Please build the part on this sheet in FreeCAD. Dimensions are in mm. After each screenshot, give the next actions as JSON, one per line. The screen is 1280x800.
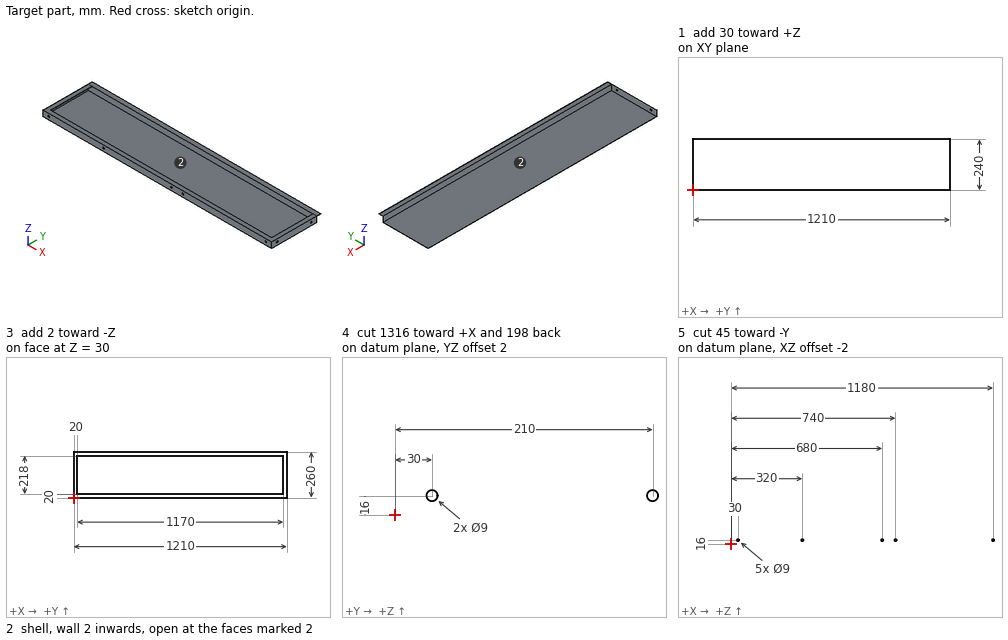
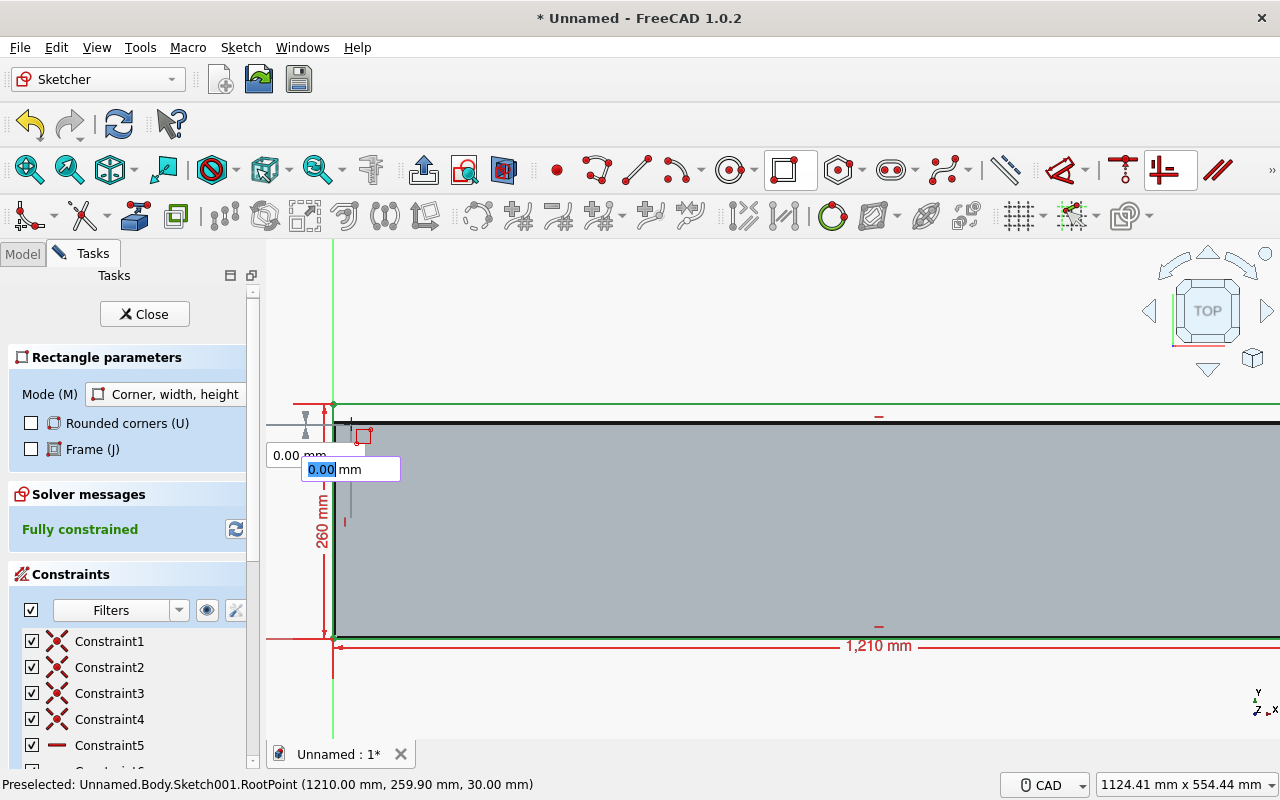
{"action": "scroll", "coordinate": [492, 449], "scroll_direction": "down", "scroll_amount": 3}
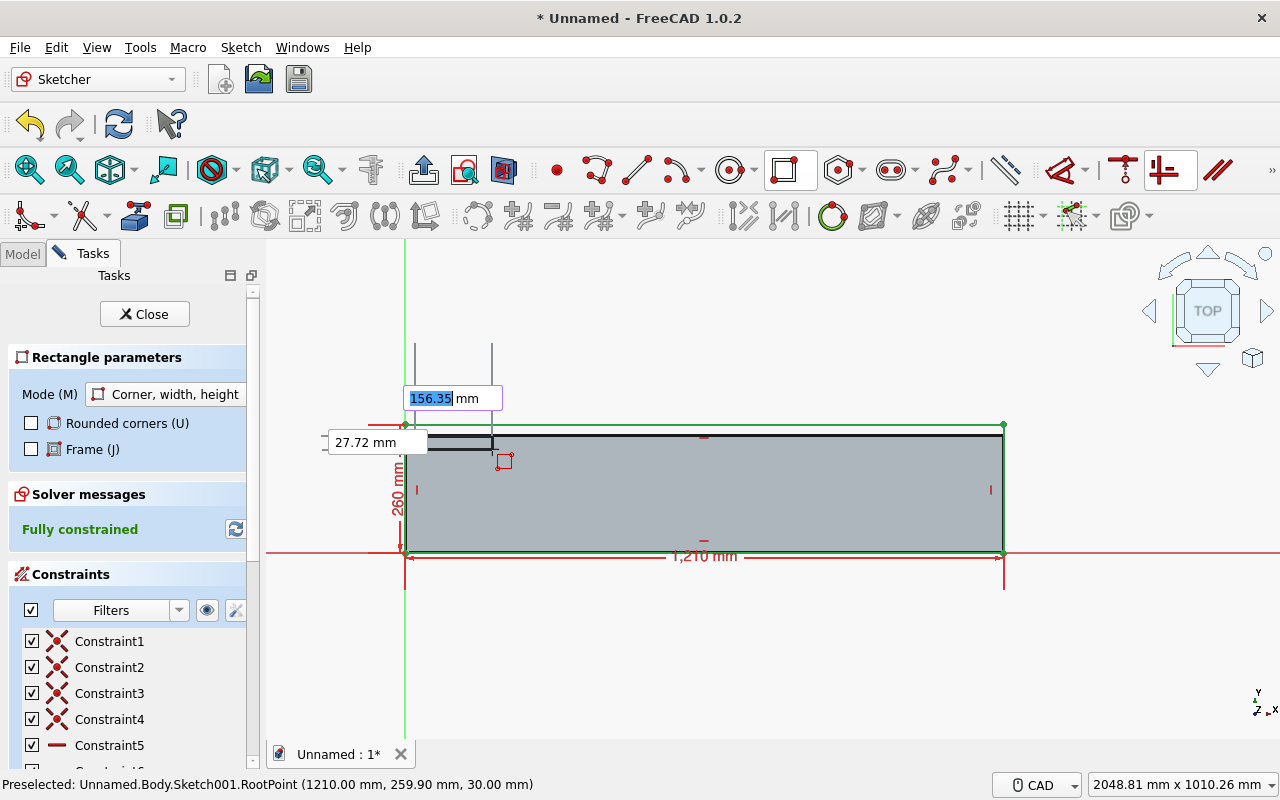
{"action": "scroll", "coordinate": [994, 543], "scroll_direction": "up", "scroll_amount": 3}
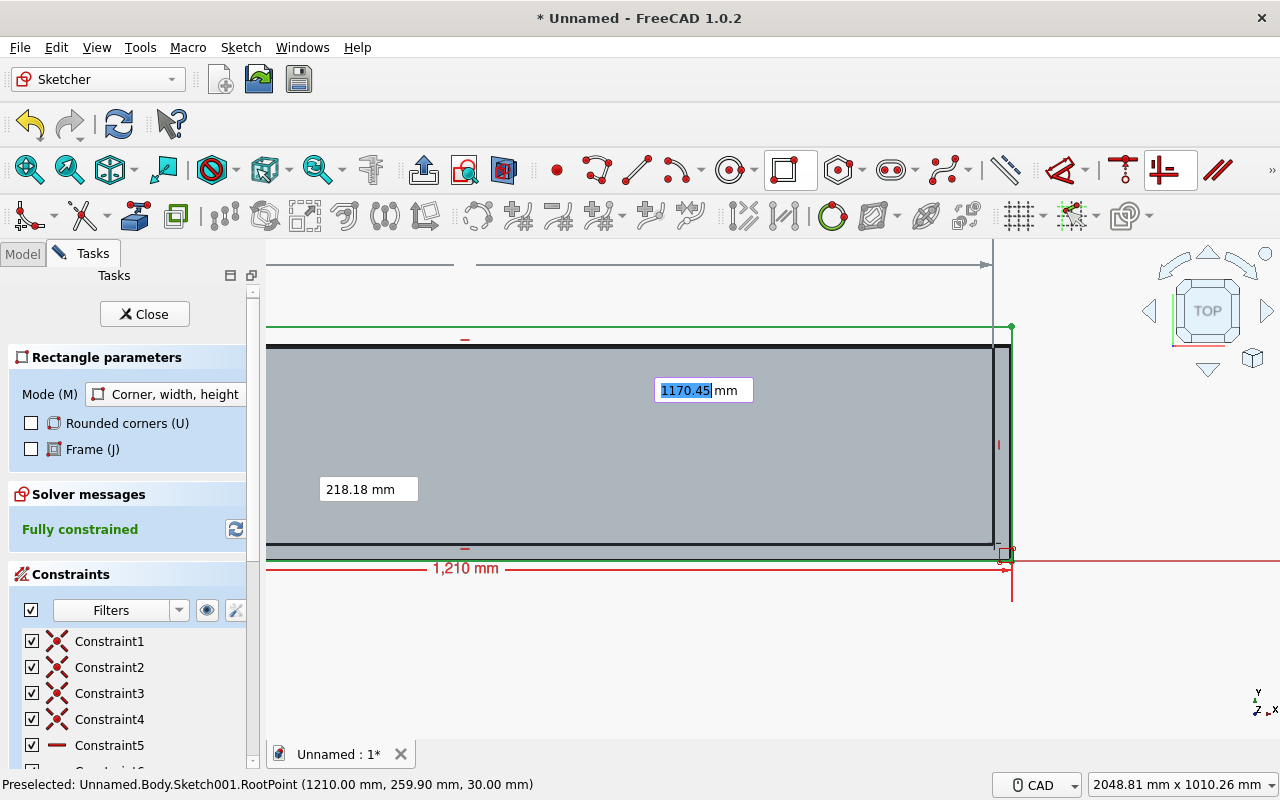
{"action": "left_click", "coordinate": [993, 543]}
{"action": "key", "text": "Escape"}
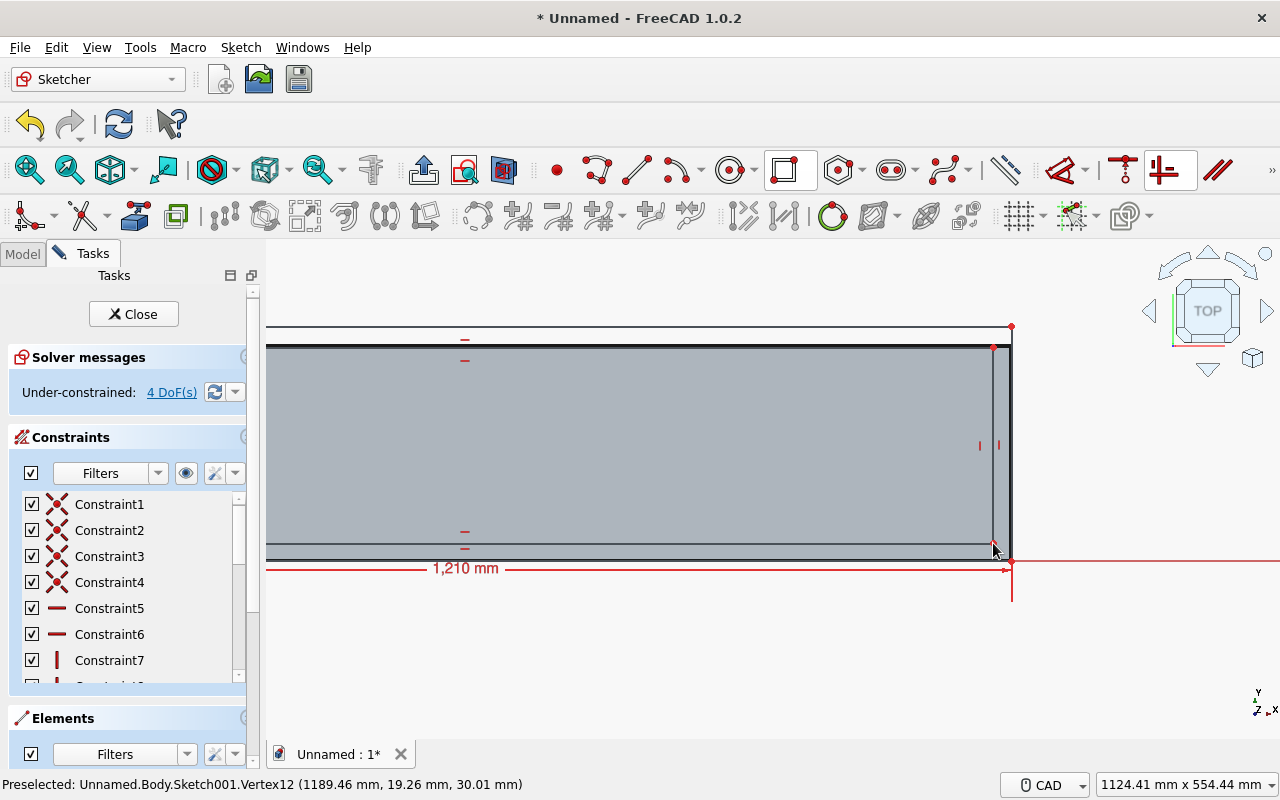
{"action": "left_click", "coordinate": [1060, 170]}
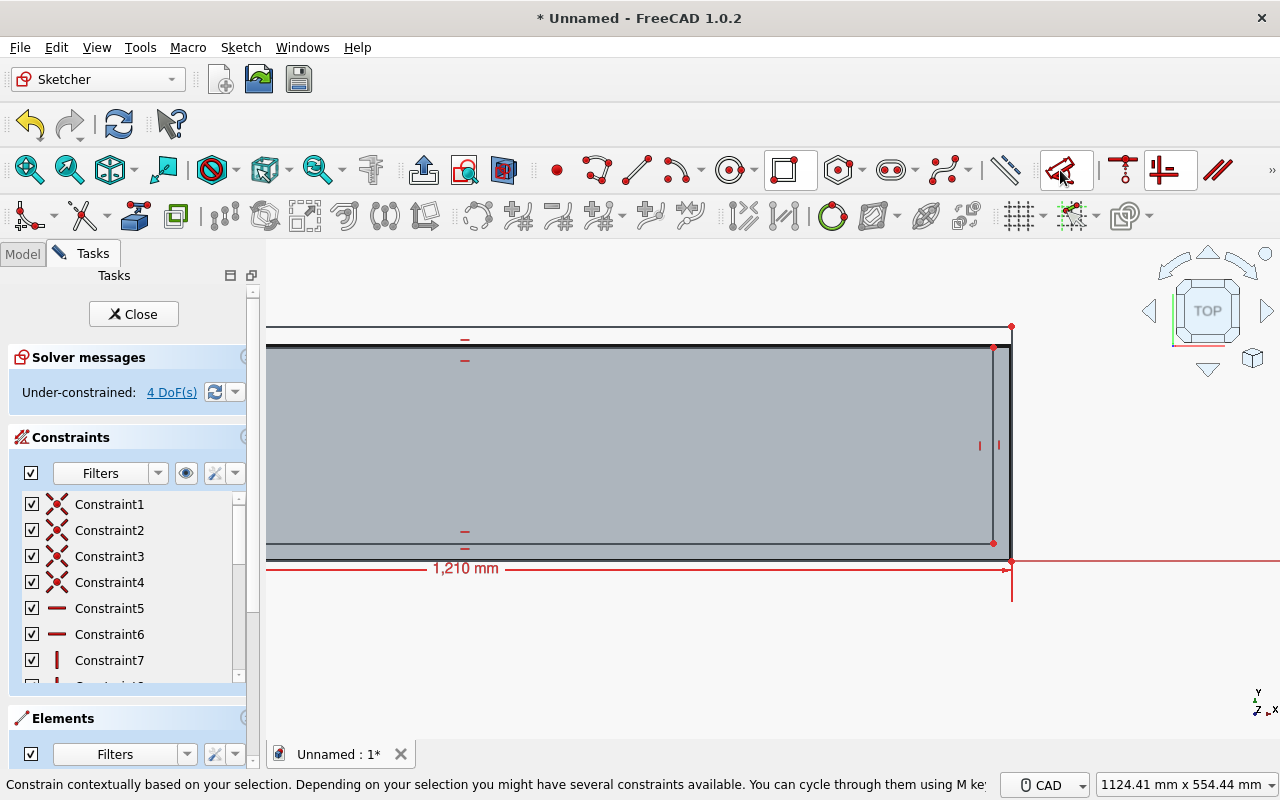
{"action": "scroll", "coordinate": [995, 544], "scroll_direction": "down", "scroll_amount": 3}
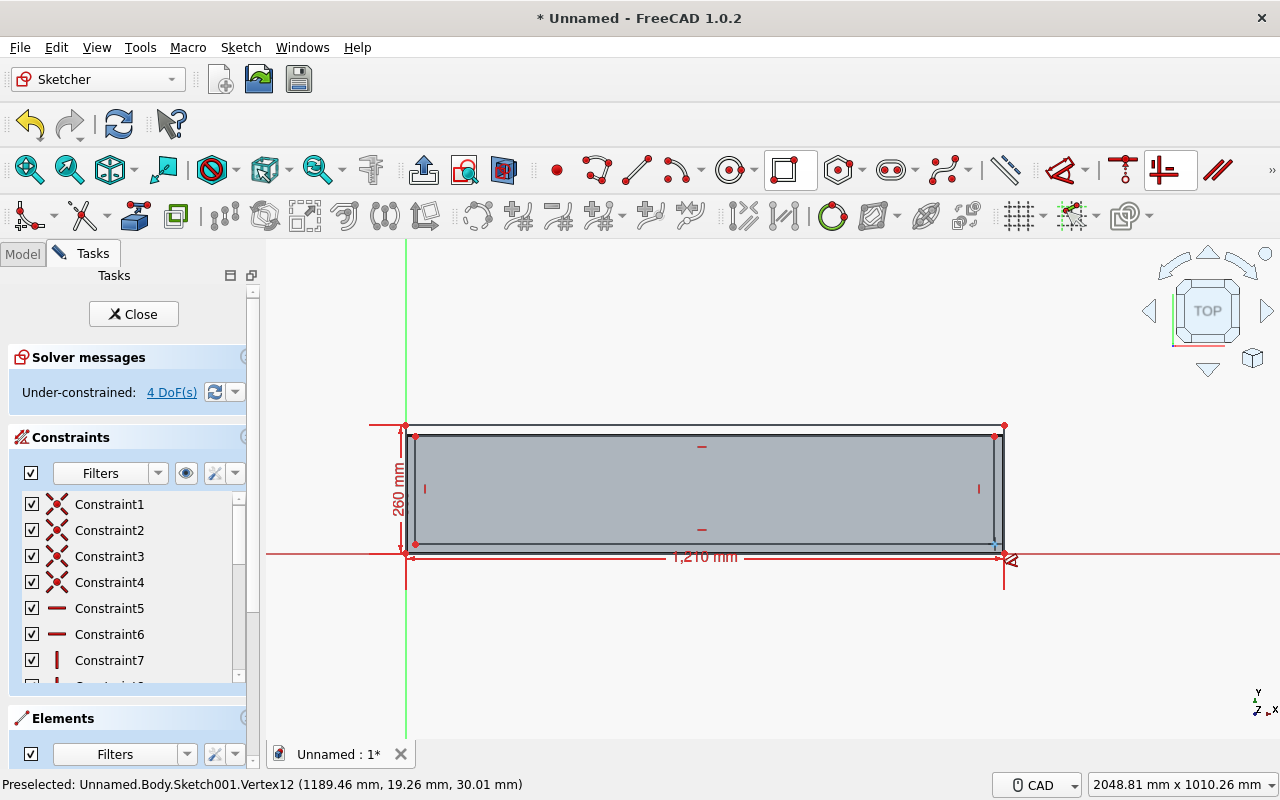
{"action": "scroll", "coordinate": [415, 469], "scroll_direction": "up", "scroll_amount": 2}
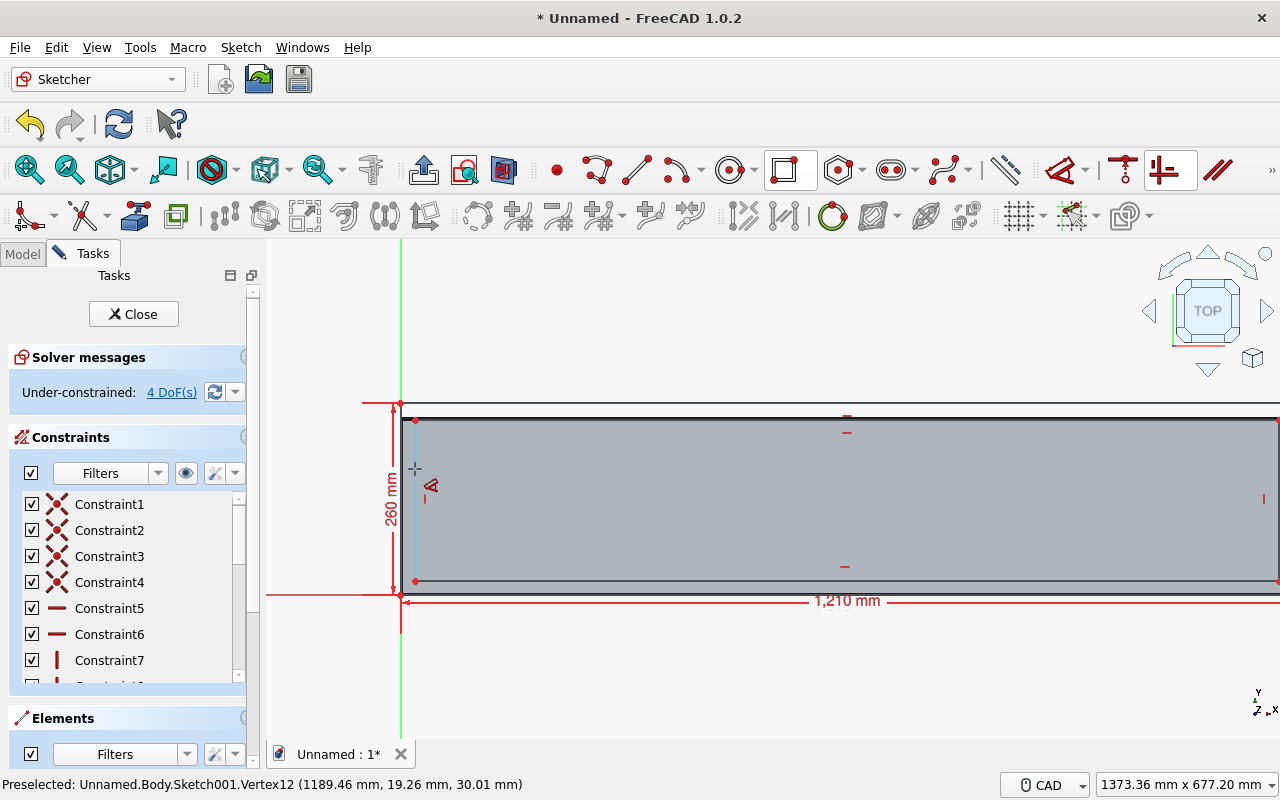
{"action": "left_click", "coordinate": [415, 468]}
{"action": "left_click", "coordinate": [381, 501]}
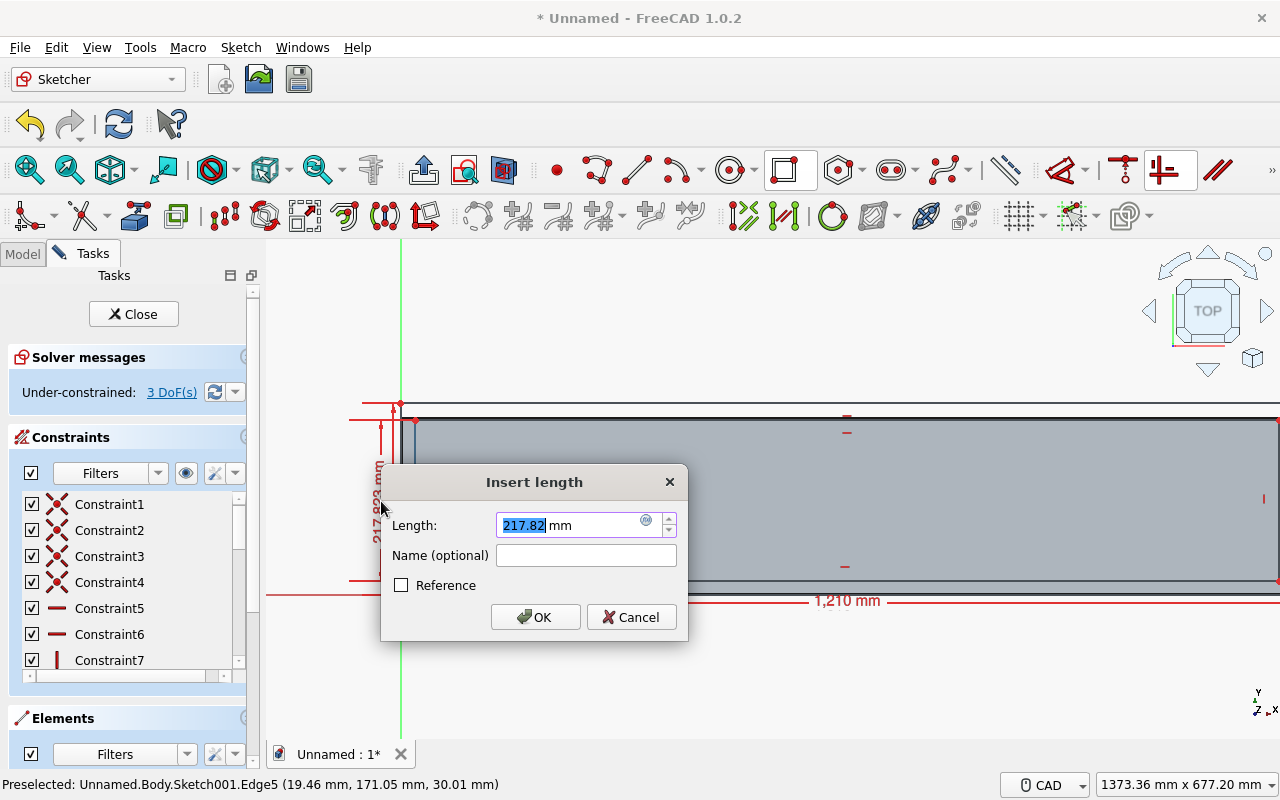
{"action": "type", "text": "218"}
{"action": "key", "text": "Return"}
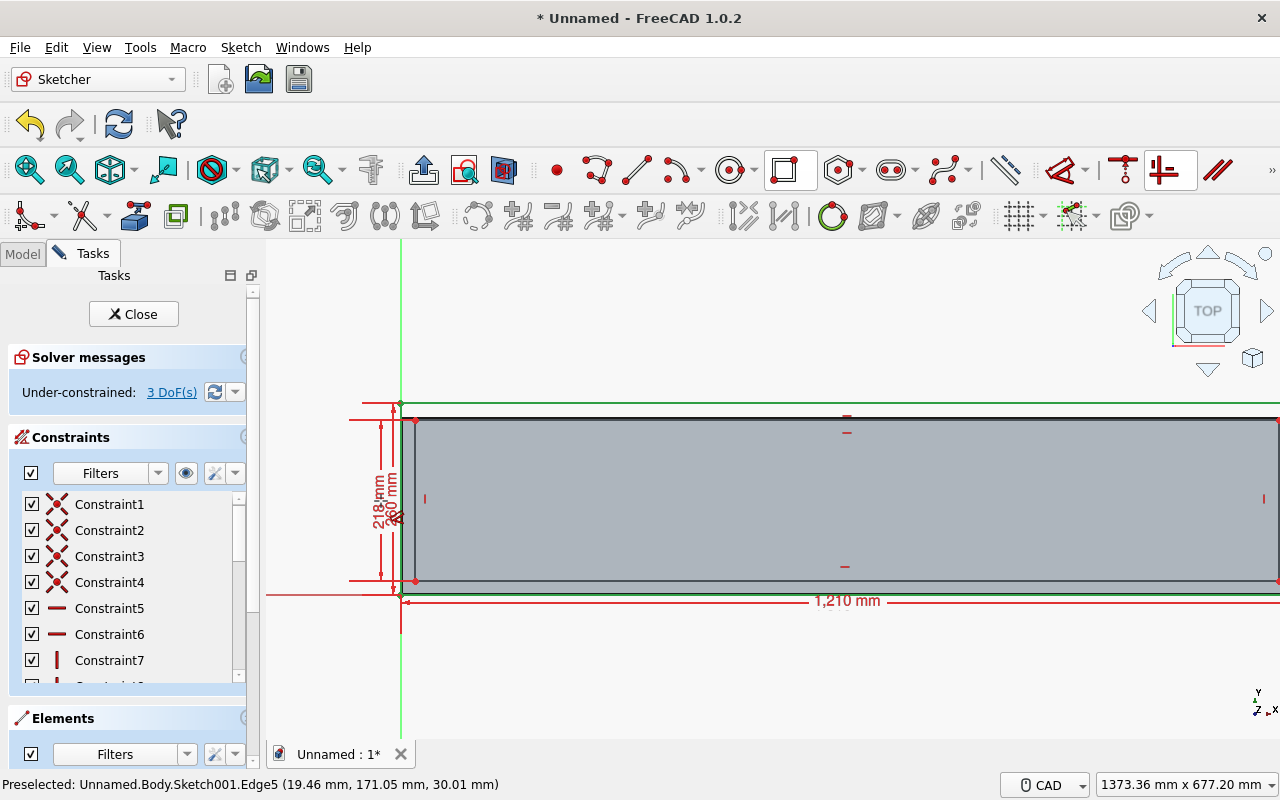
{"action": "scroll", "coordinate": [415, 420], "scroll_direction": "up", "scroll_amount": 5}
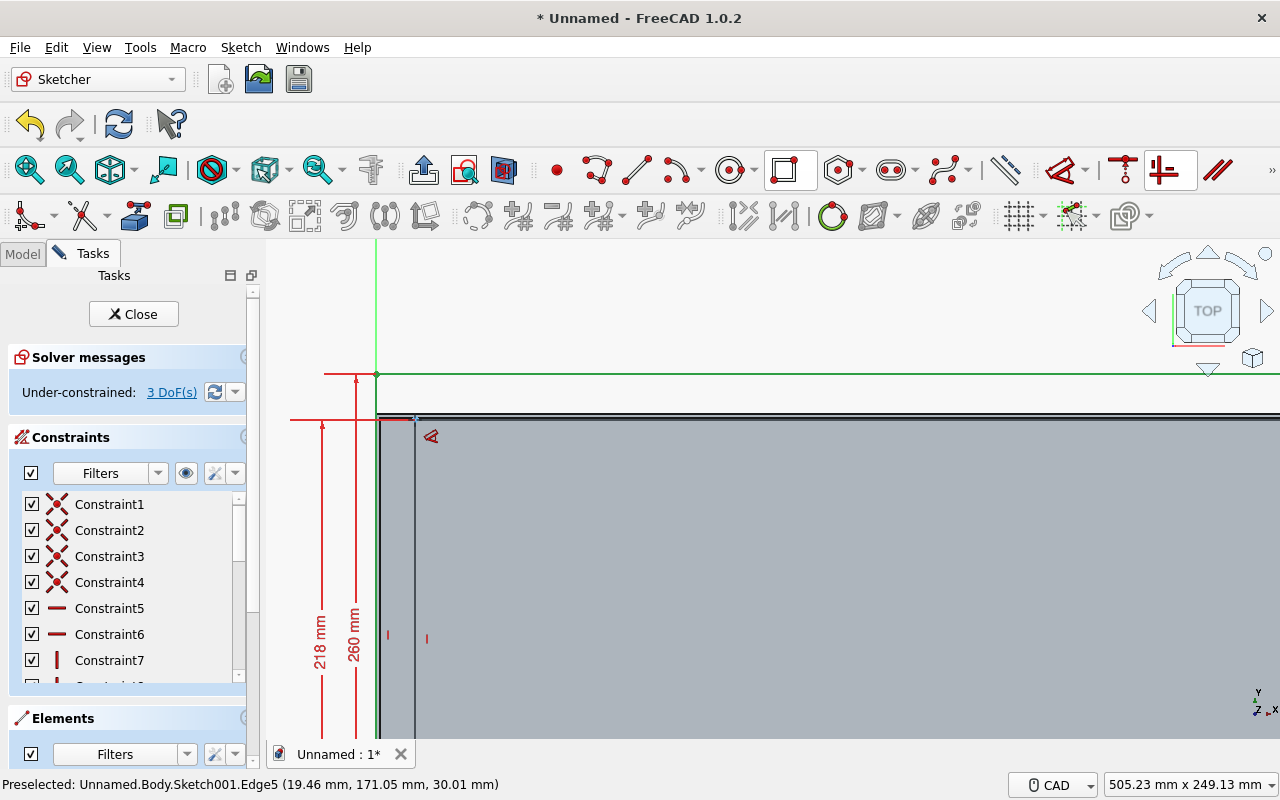
{"action": "left_click", "coordinate": [415, 420]}
{"action": "left_click", "coordinate": [396, 338]}